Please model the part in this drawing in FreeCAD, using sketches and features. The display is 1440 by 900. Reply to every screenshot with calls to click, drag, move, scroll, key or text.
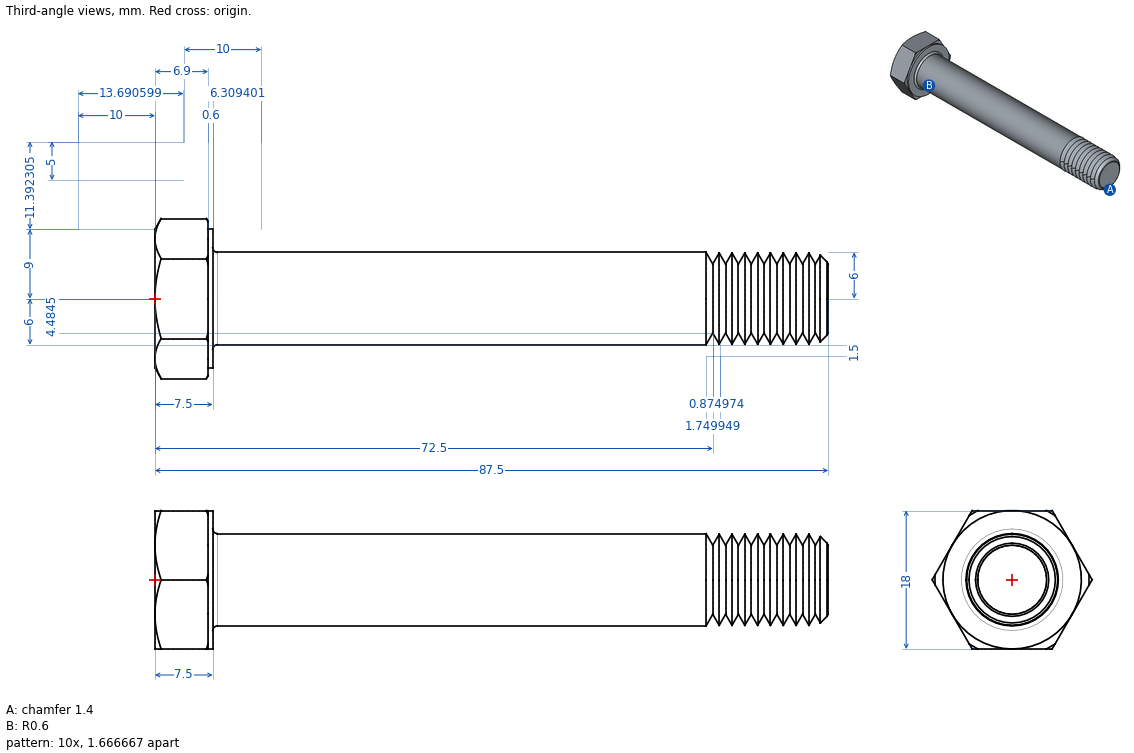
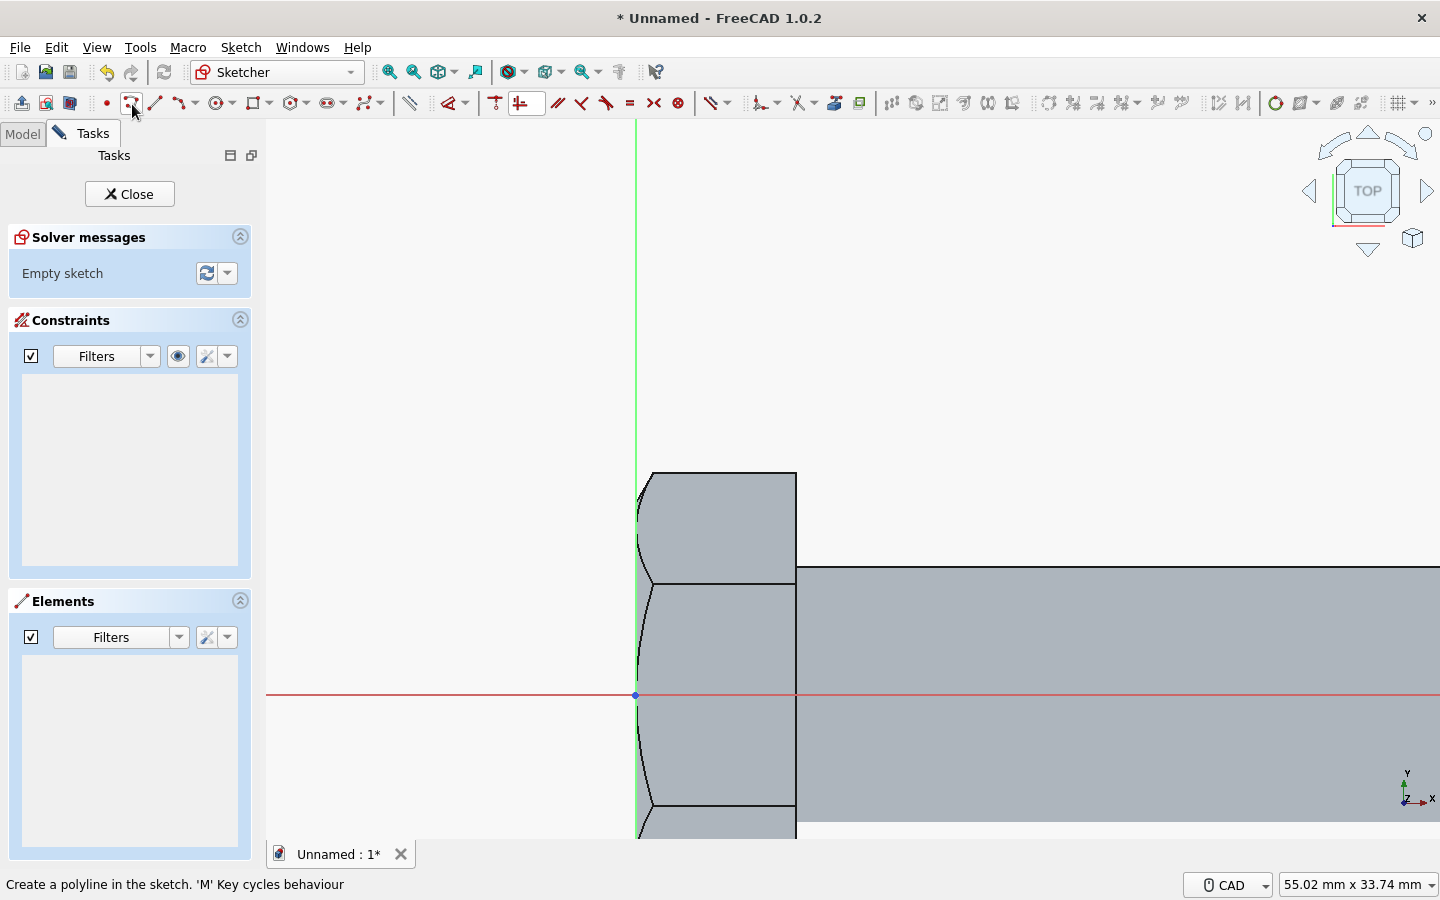
click(796, 503)
click(931, 503)
click(931, 260)
click(717, 260)
click(717, 367)
click(796, 504)
key(Escape)
key(Escape)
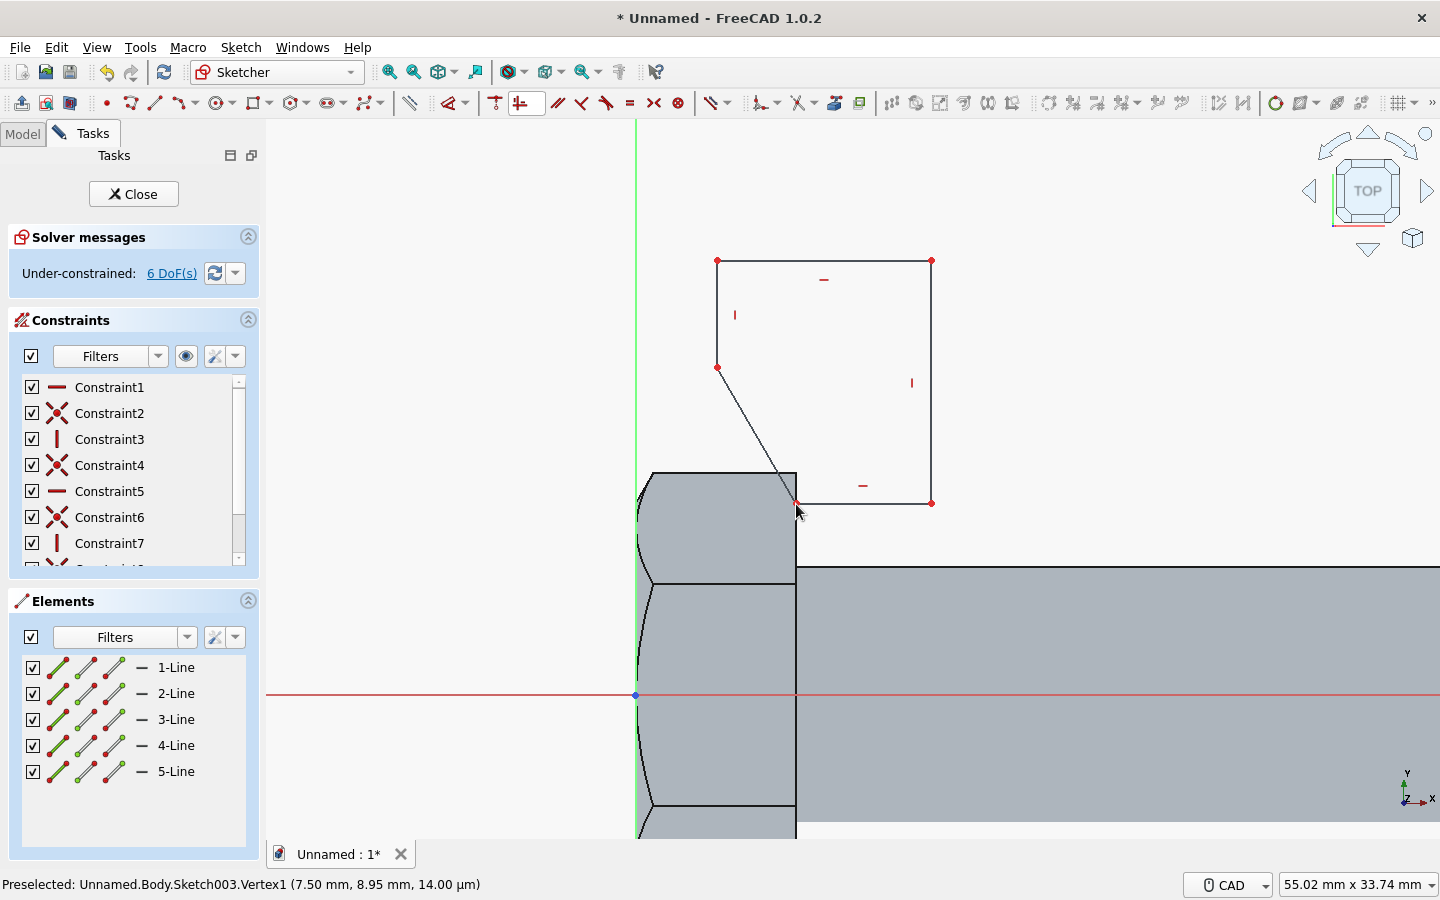
click(448, 104)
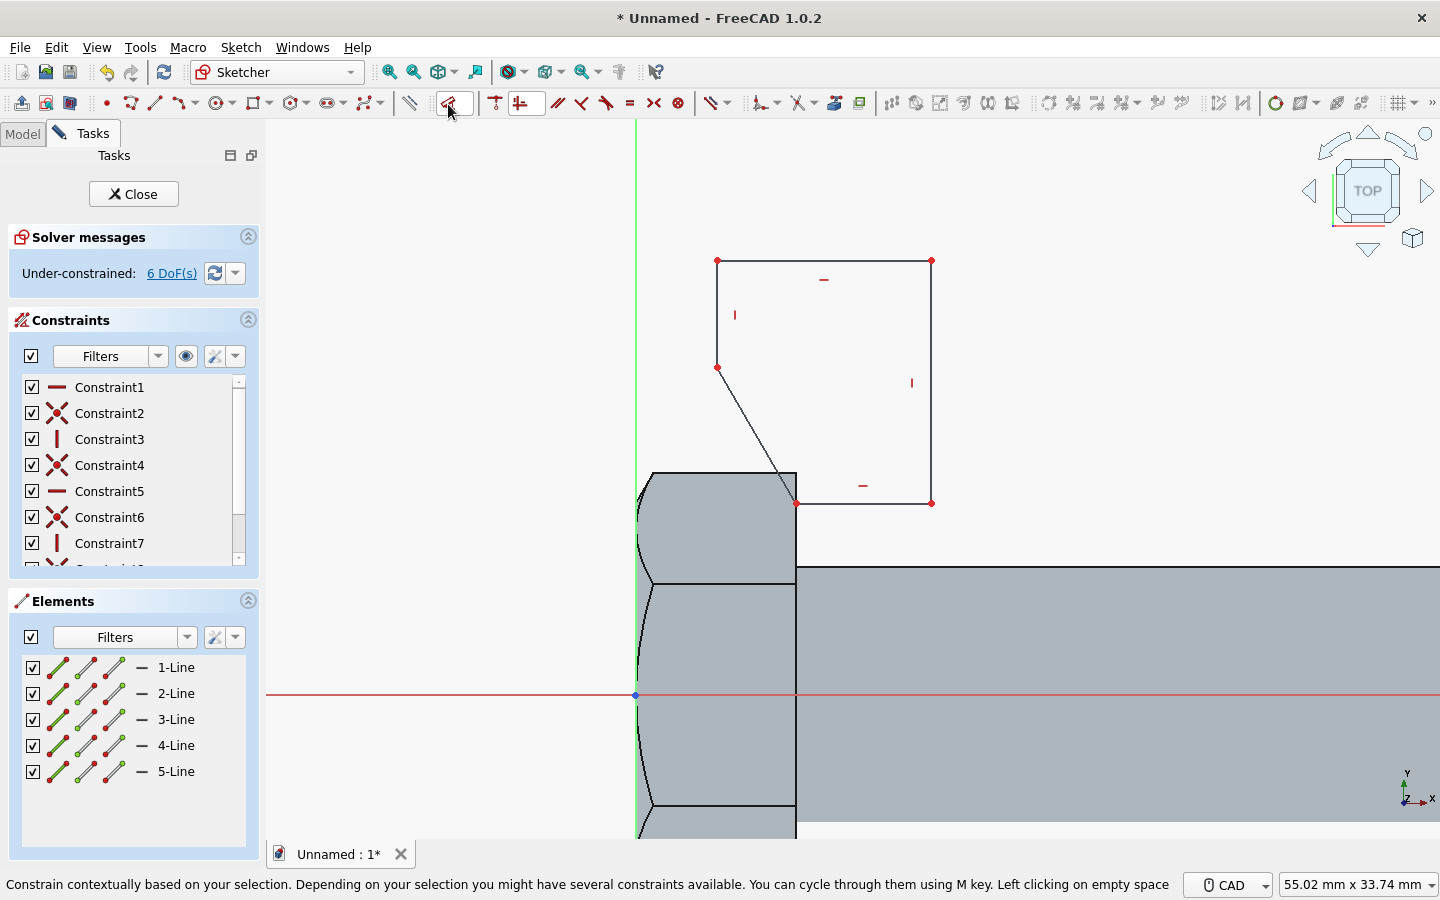
click(717, 293)
click(683, 315)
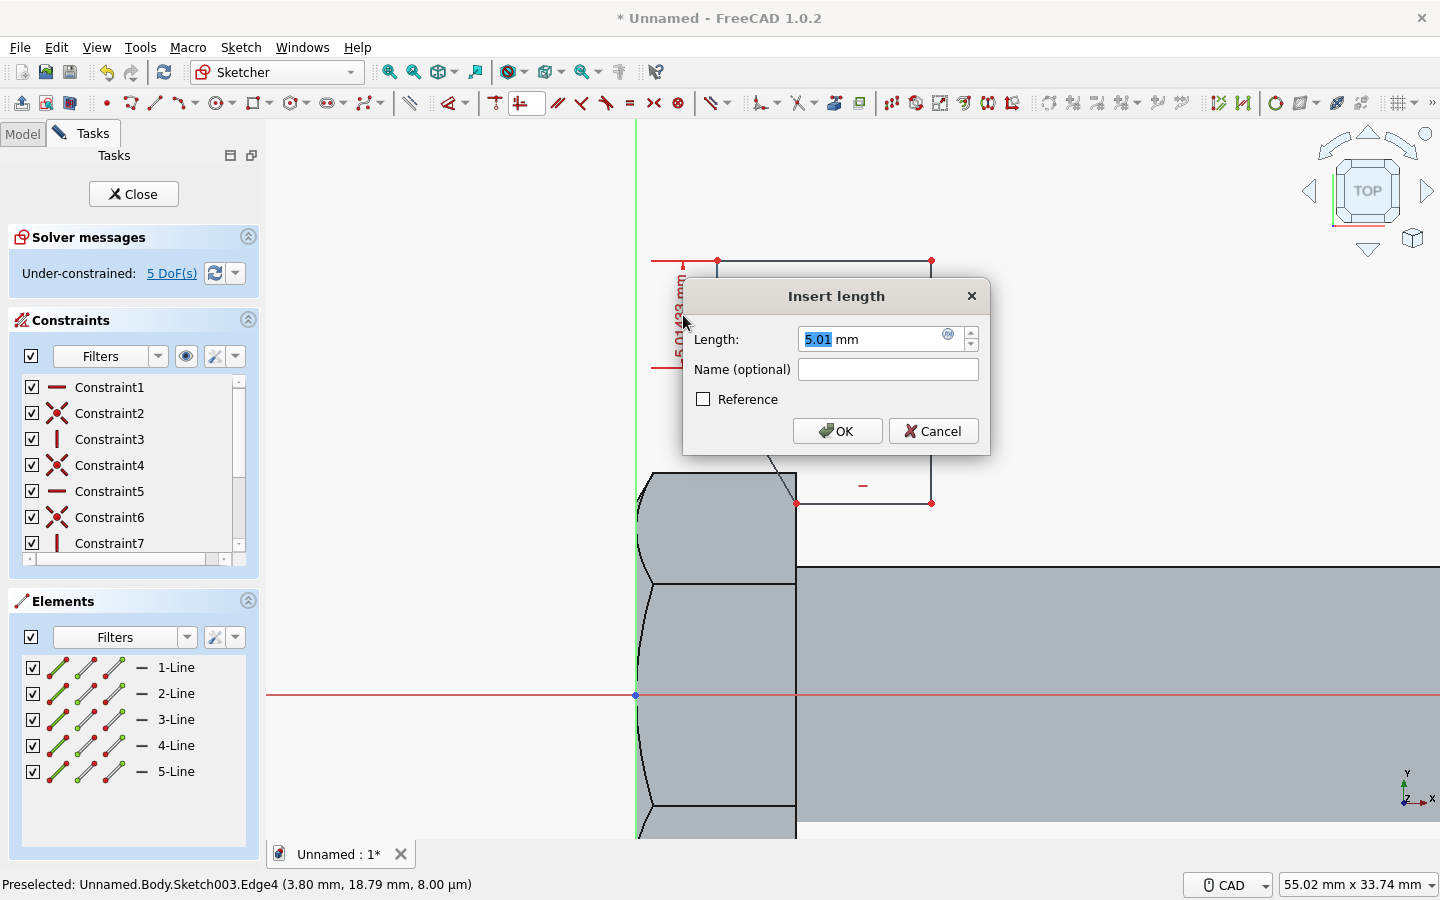
text(5)
key(Return)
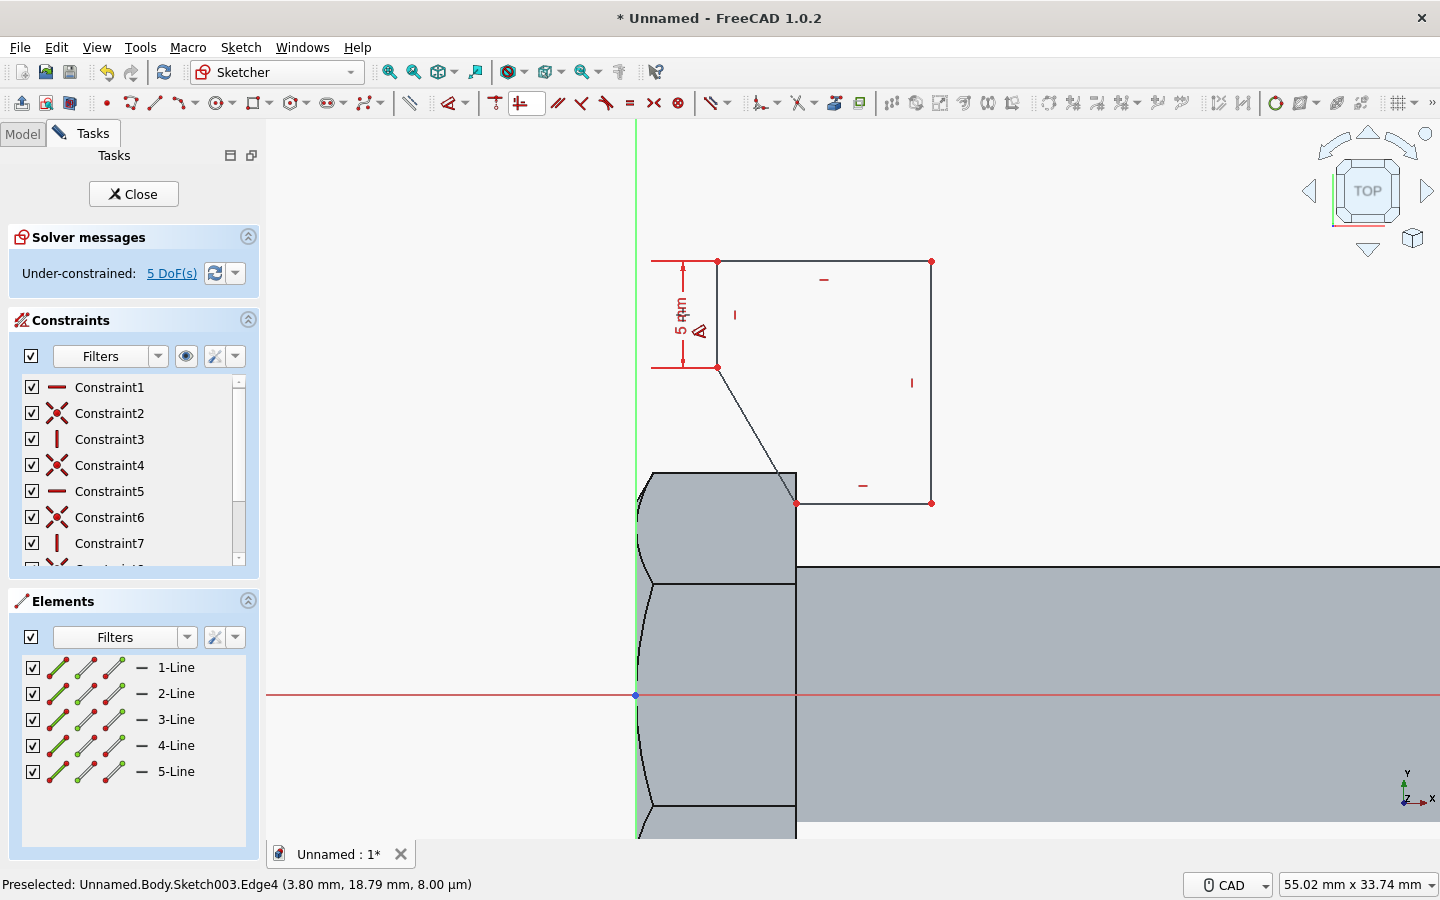
click(867, 261)
click(824, 227)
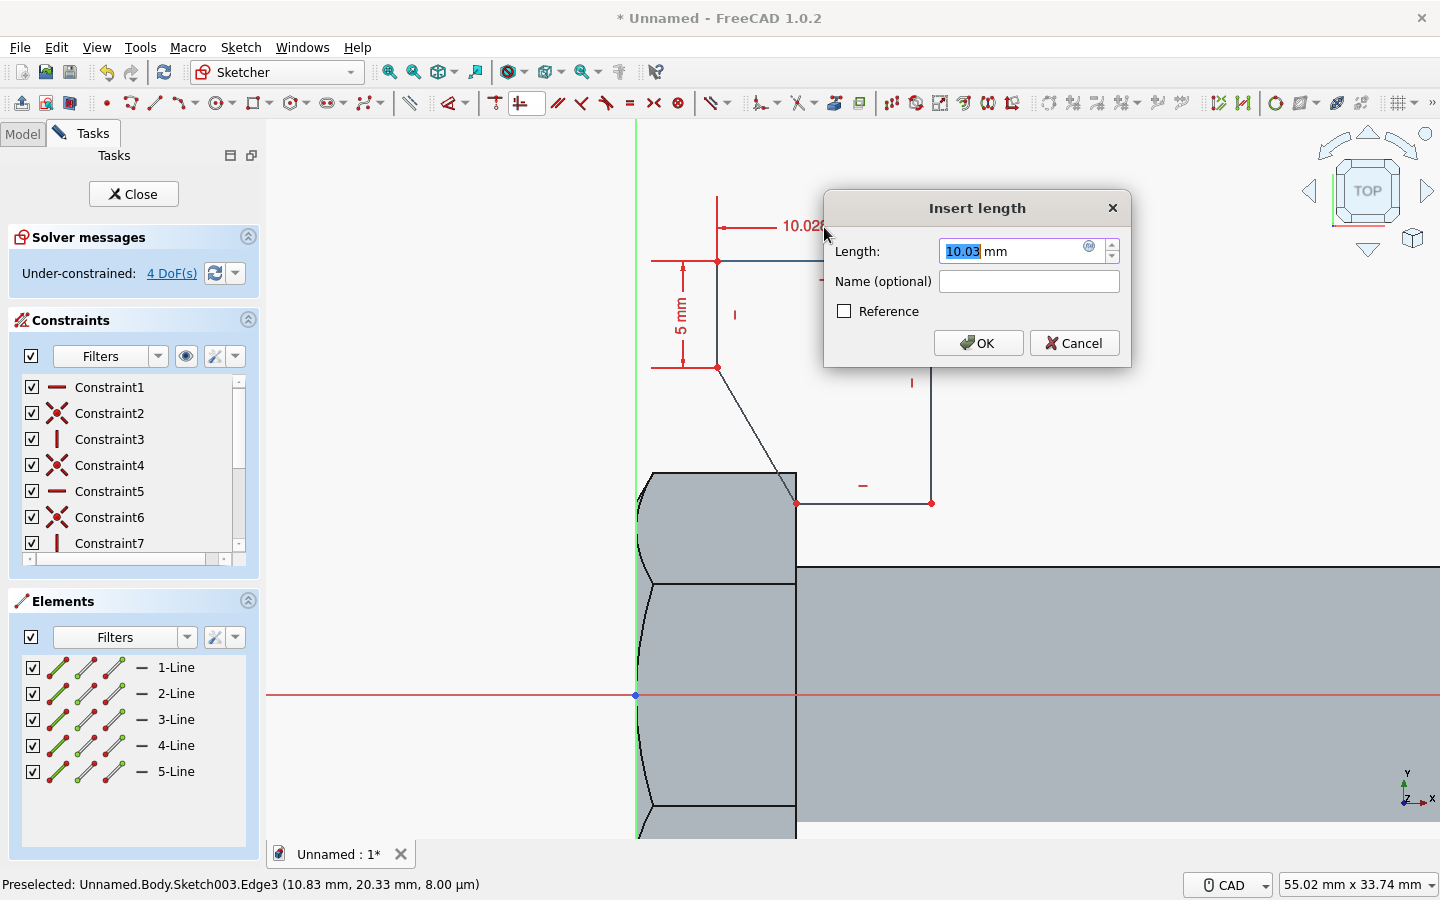
text(10)
key(Return)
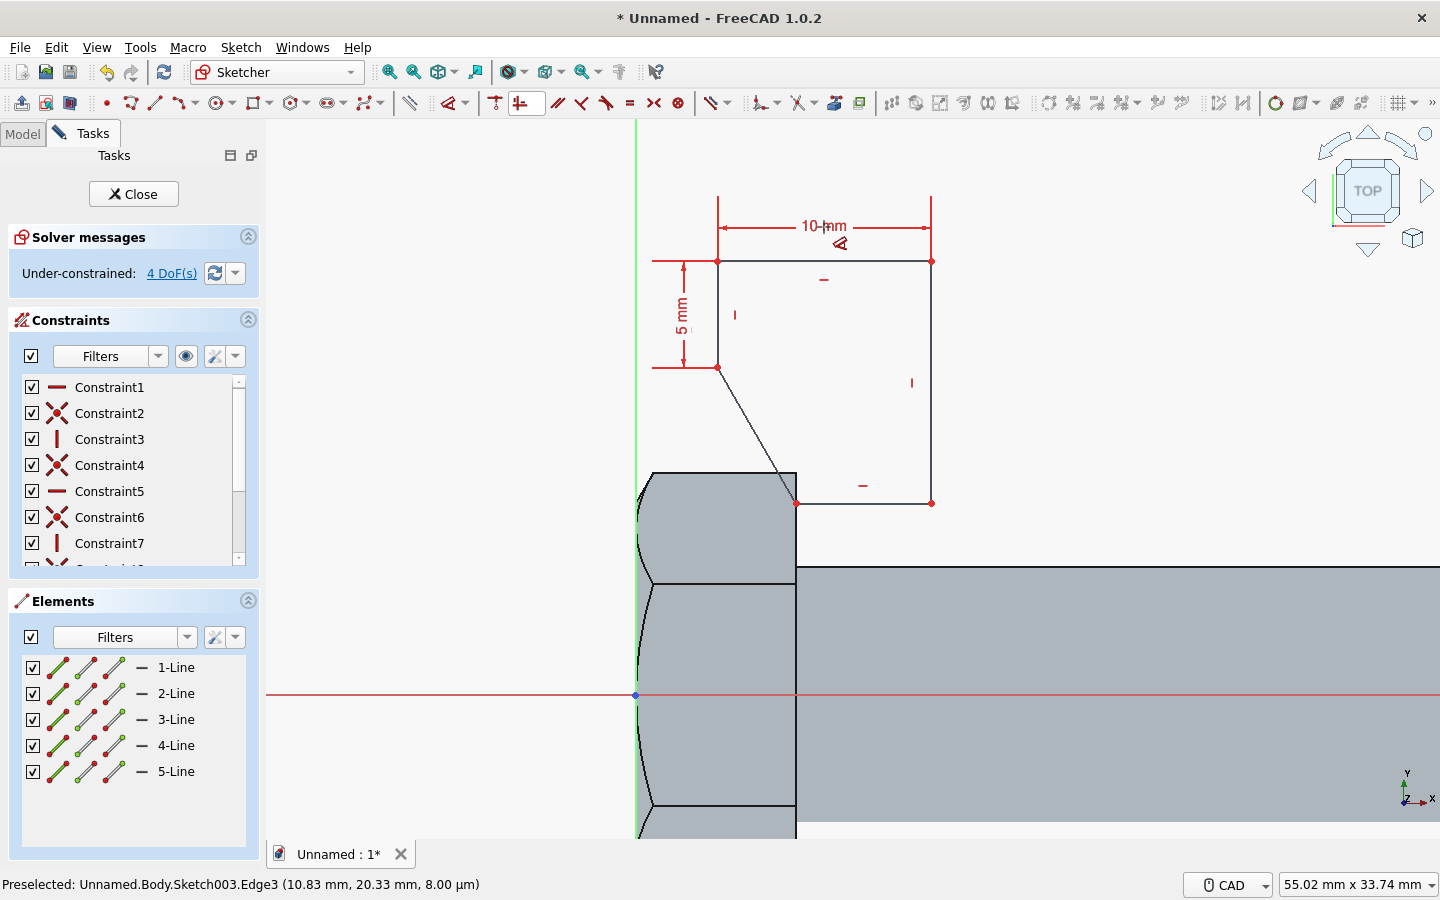
click(796, 504)
click(602, 600)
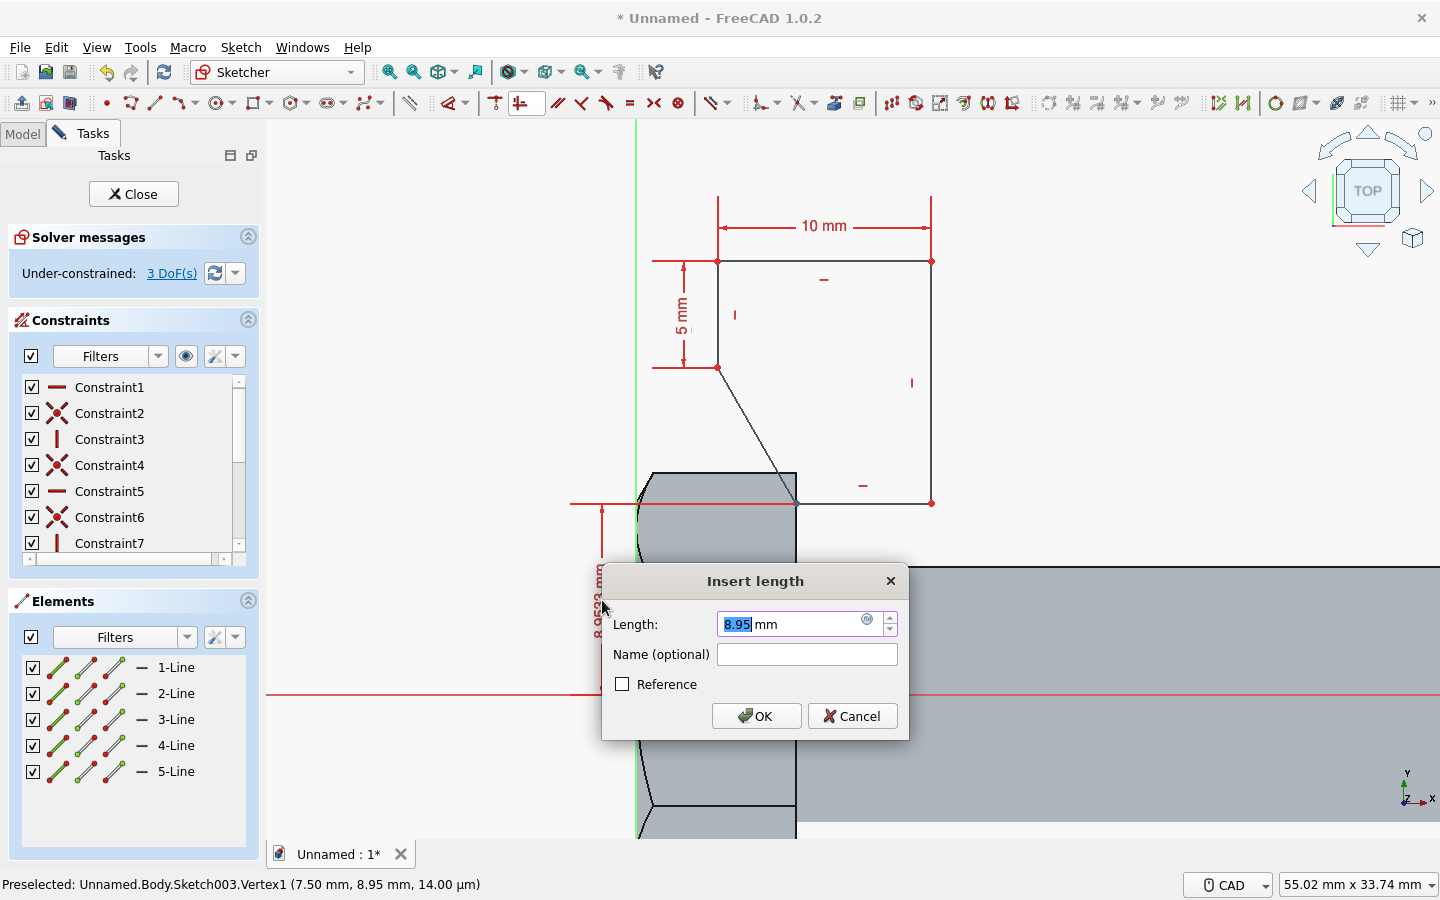
text(9)
key(Return)